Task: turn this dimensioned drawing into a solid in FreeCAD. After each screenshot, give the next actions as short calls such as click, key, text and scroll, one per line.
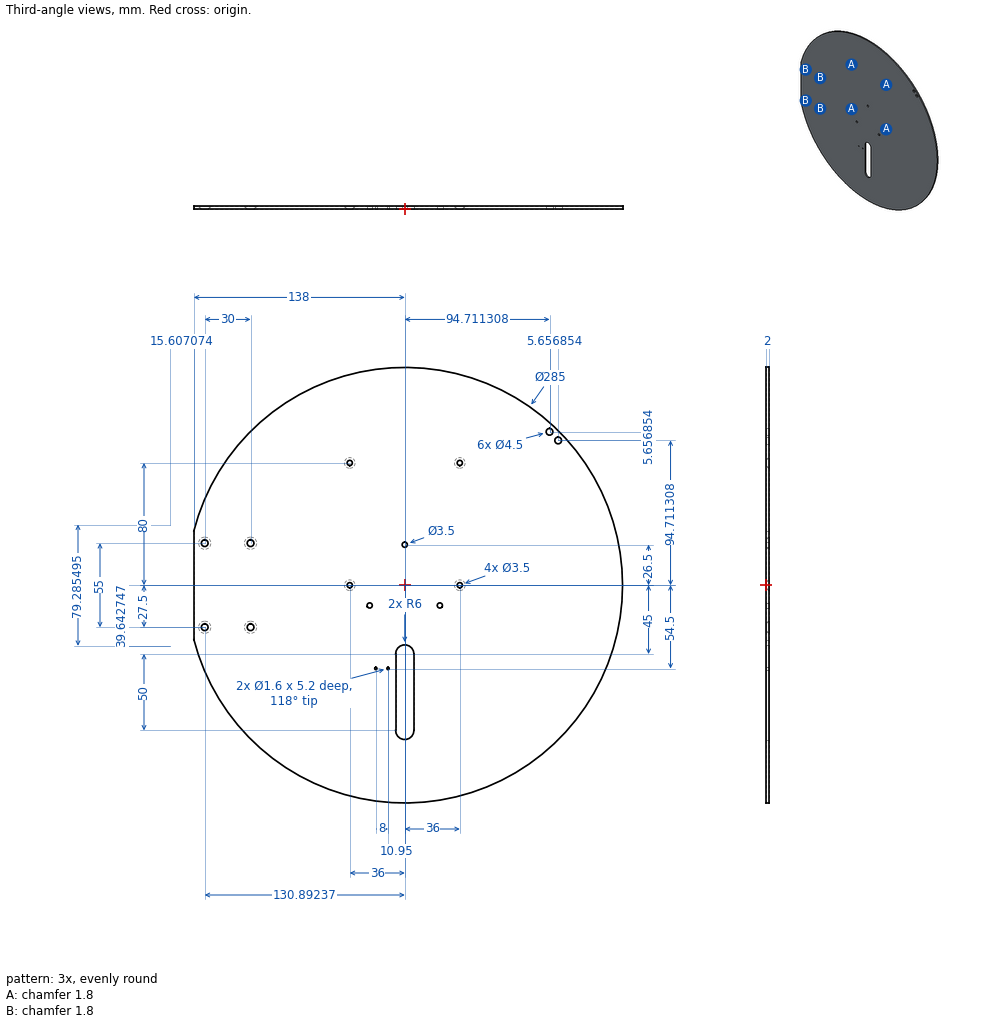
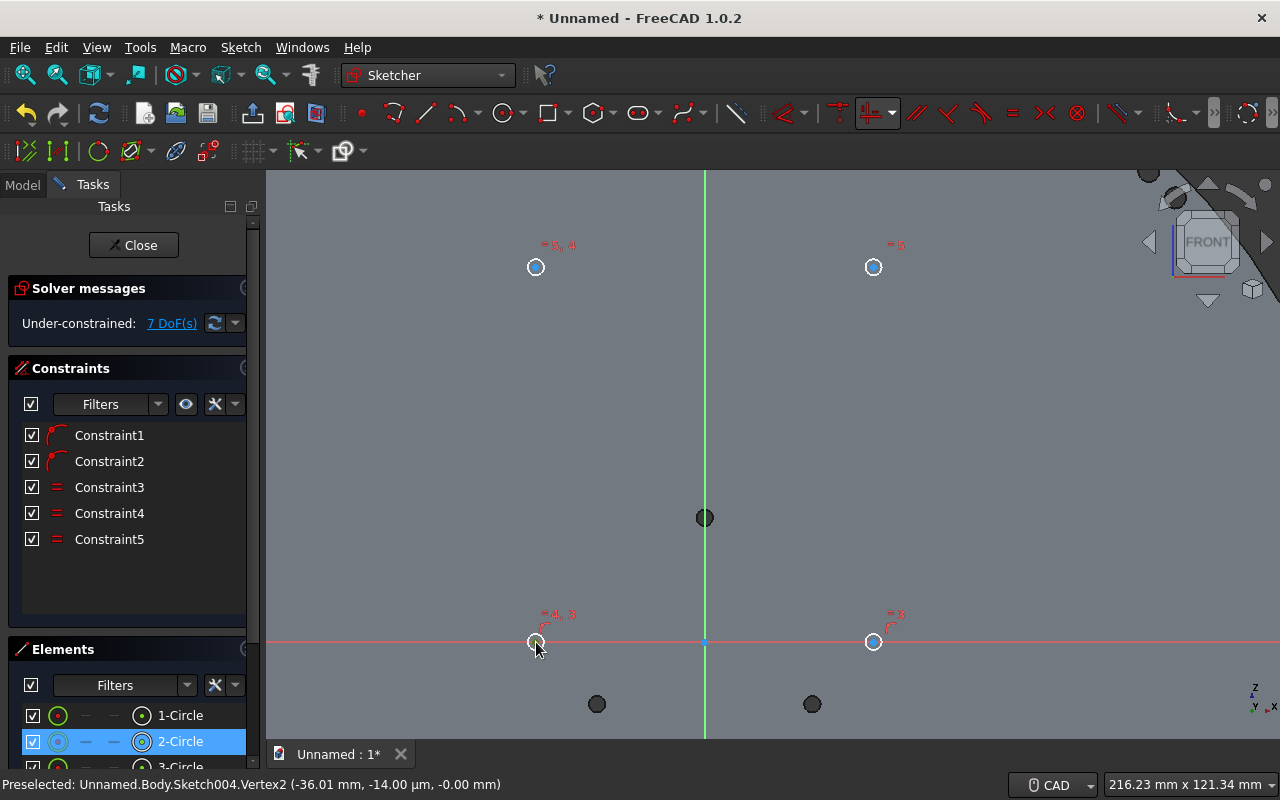
click(536, 267)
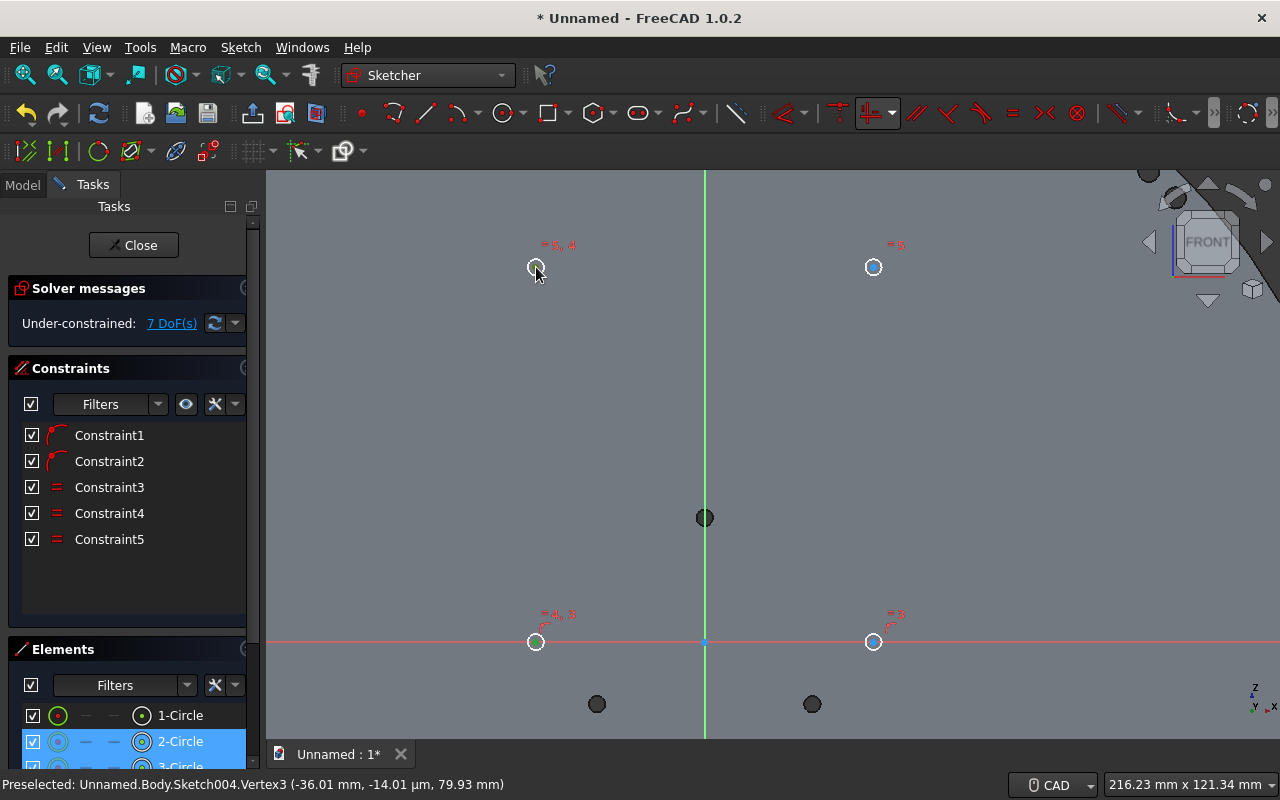
click(894, 114)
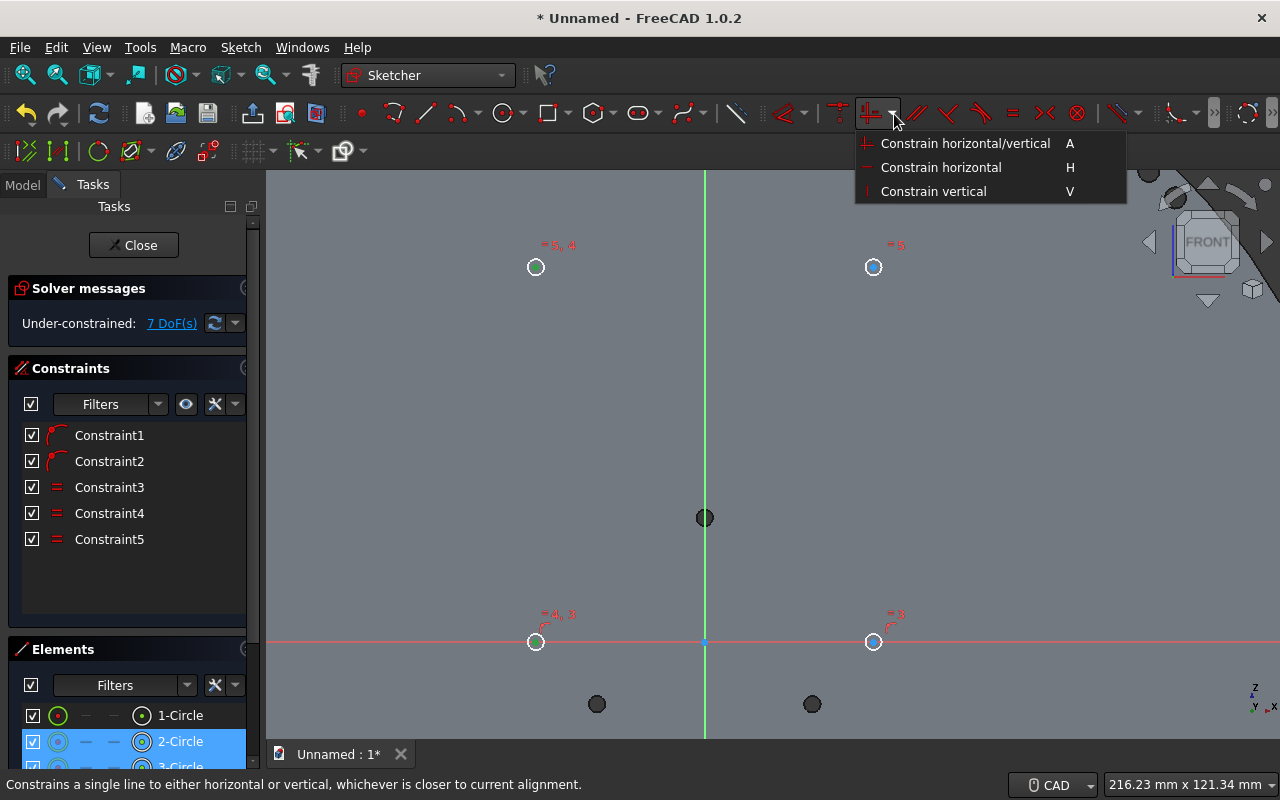
click(991, 191)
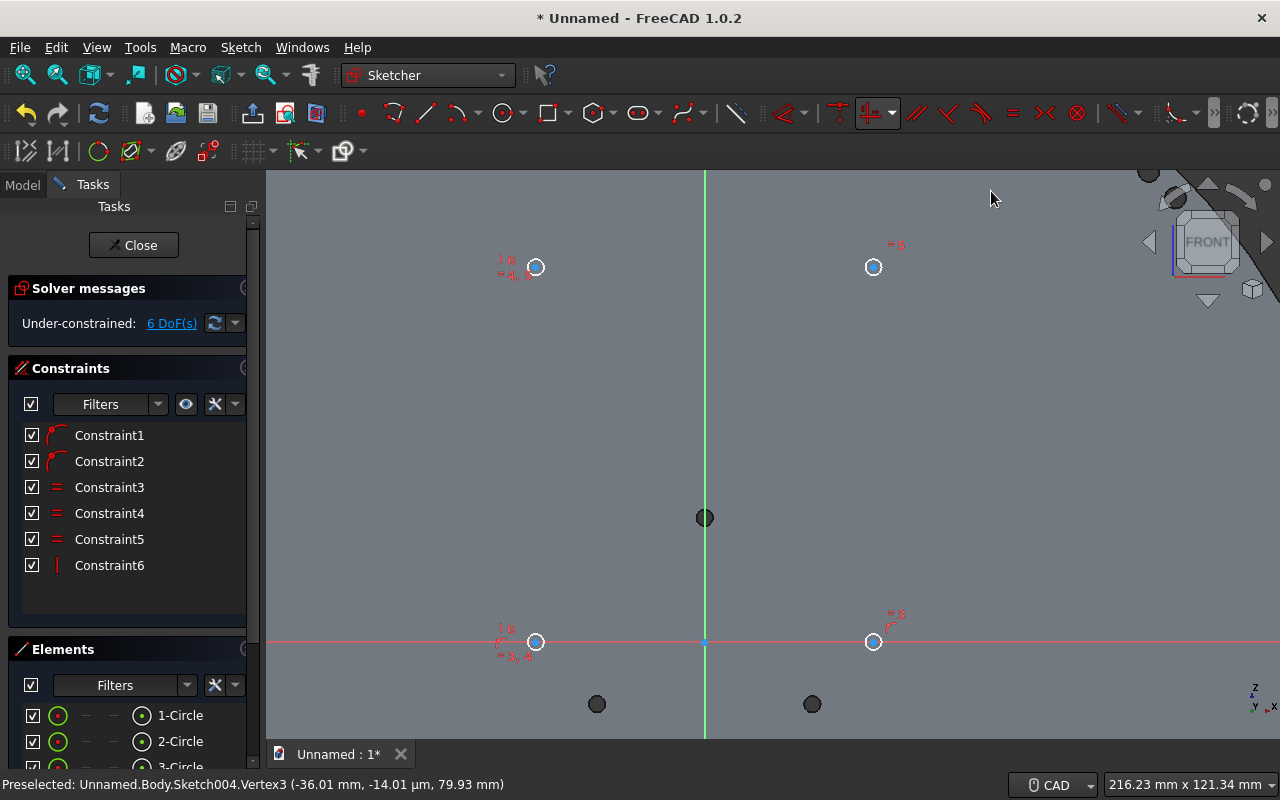
click(874, 642)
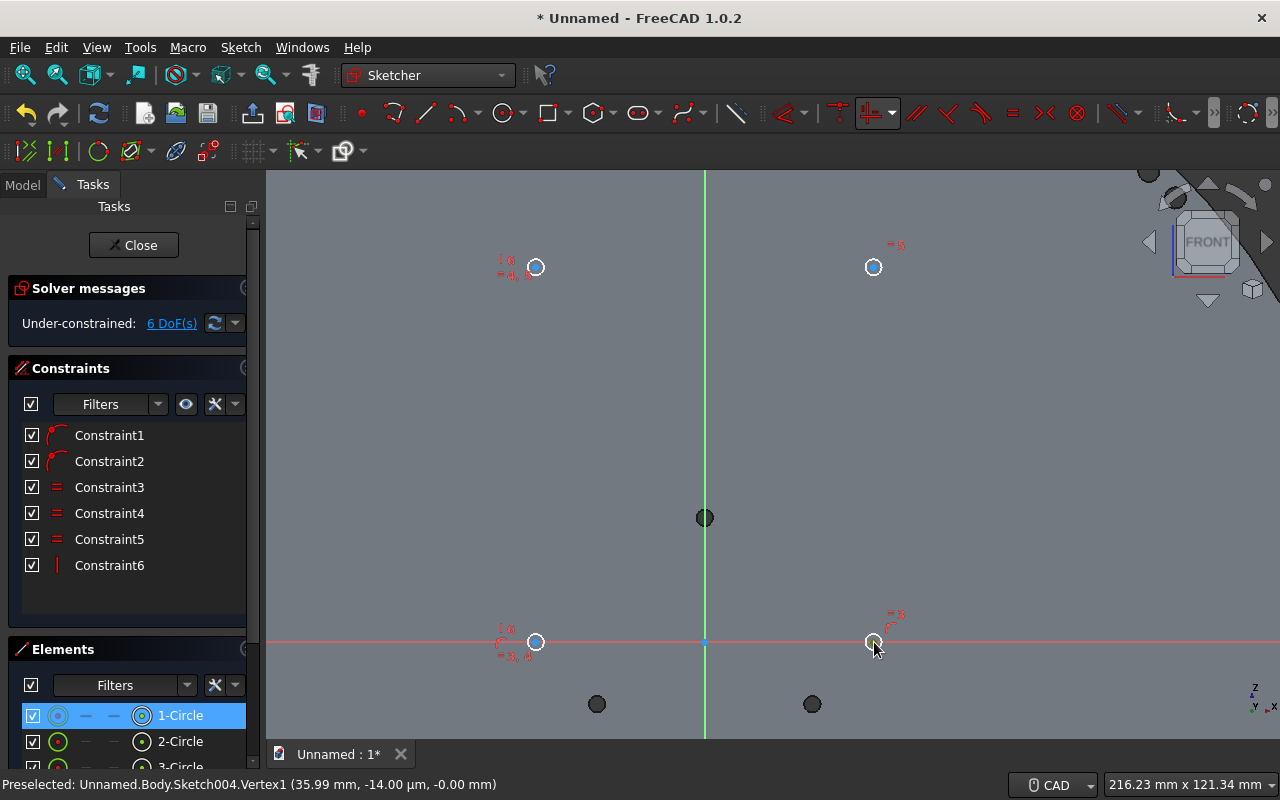
click(874, 267)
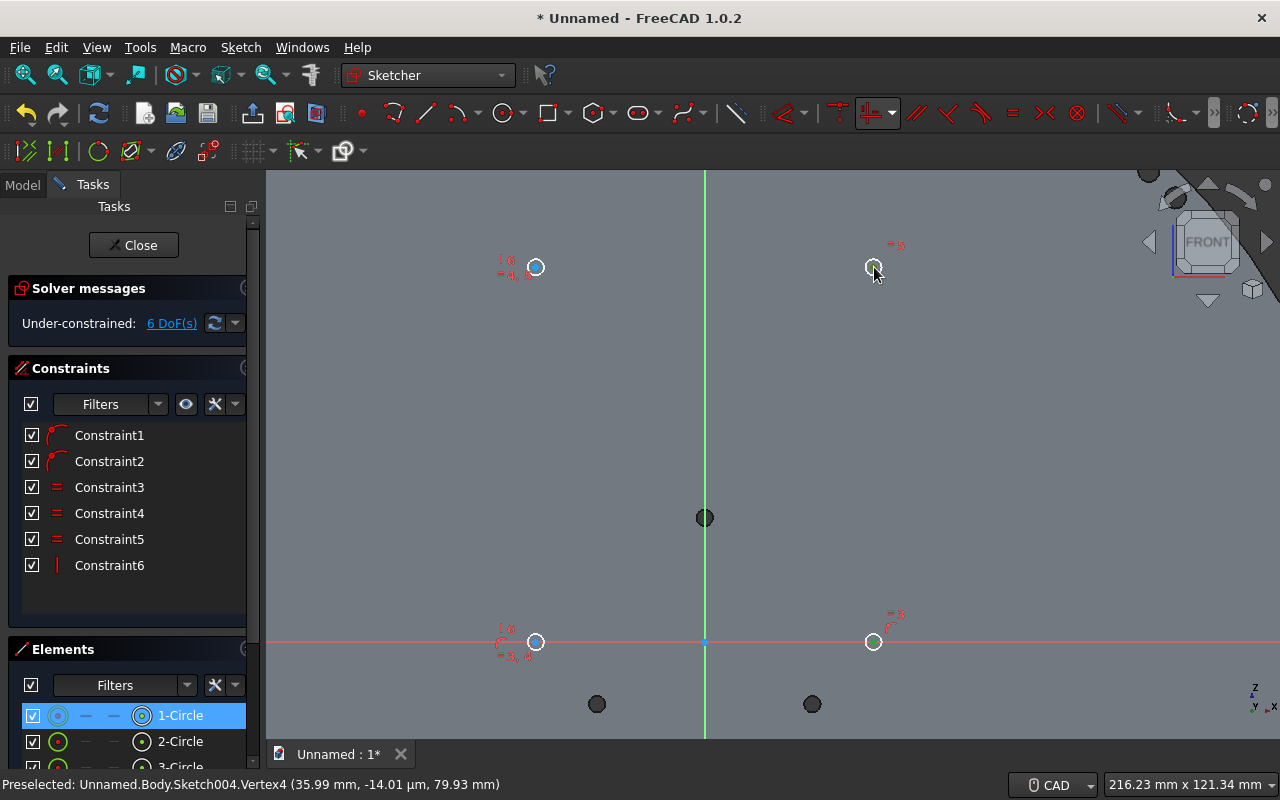
click(894, 114)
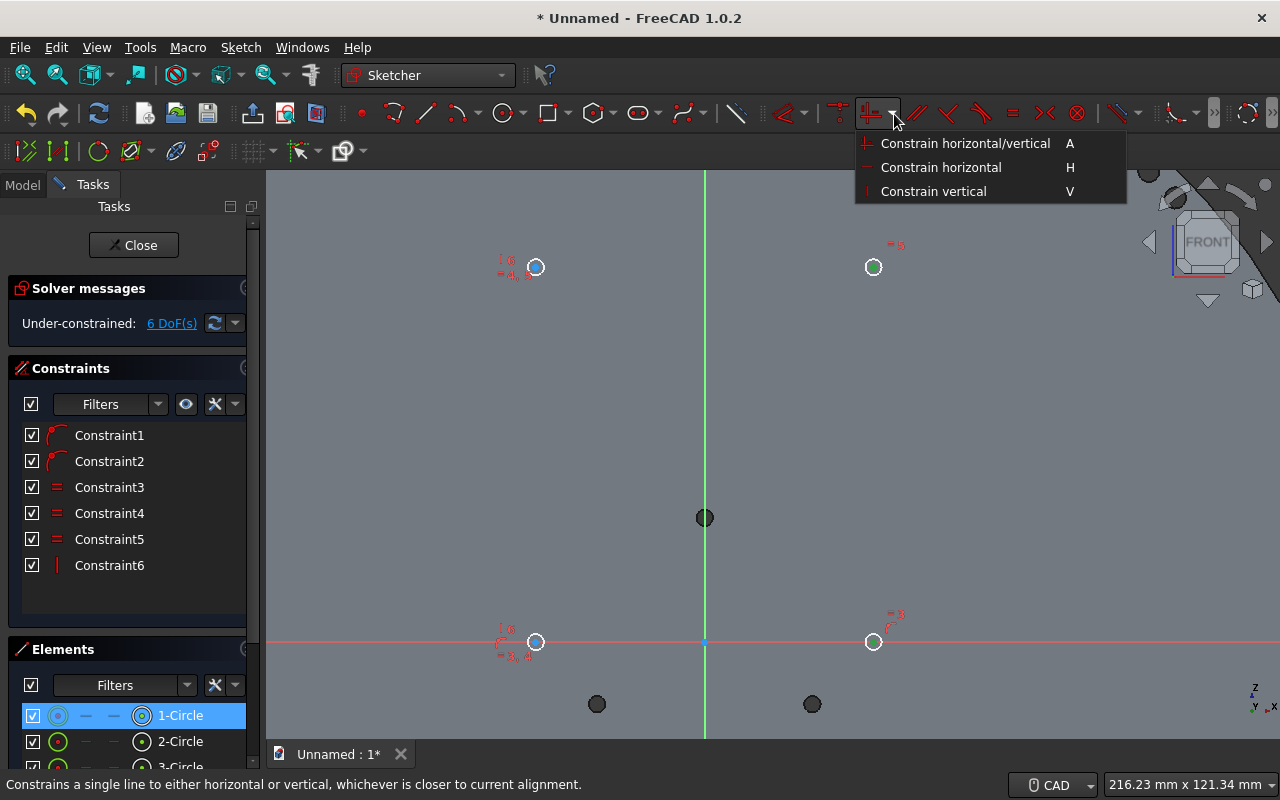
click(991, 191)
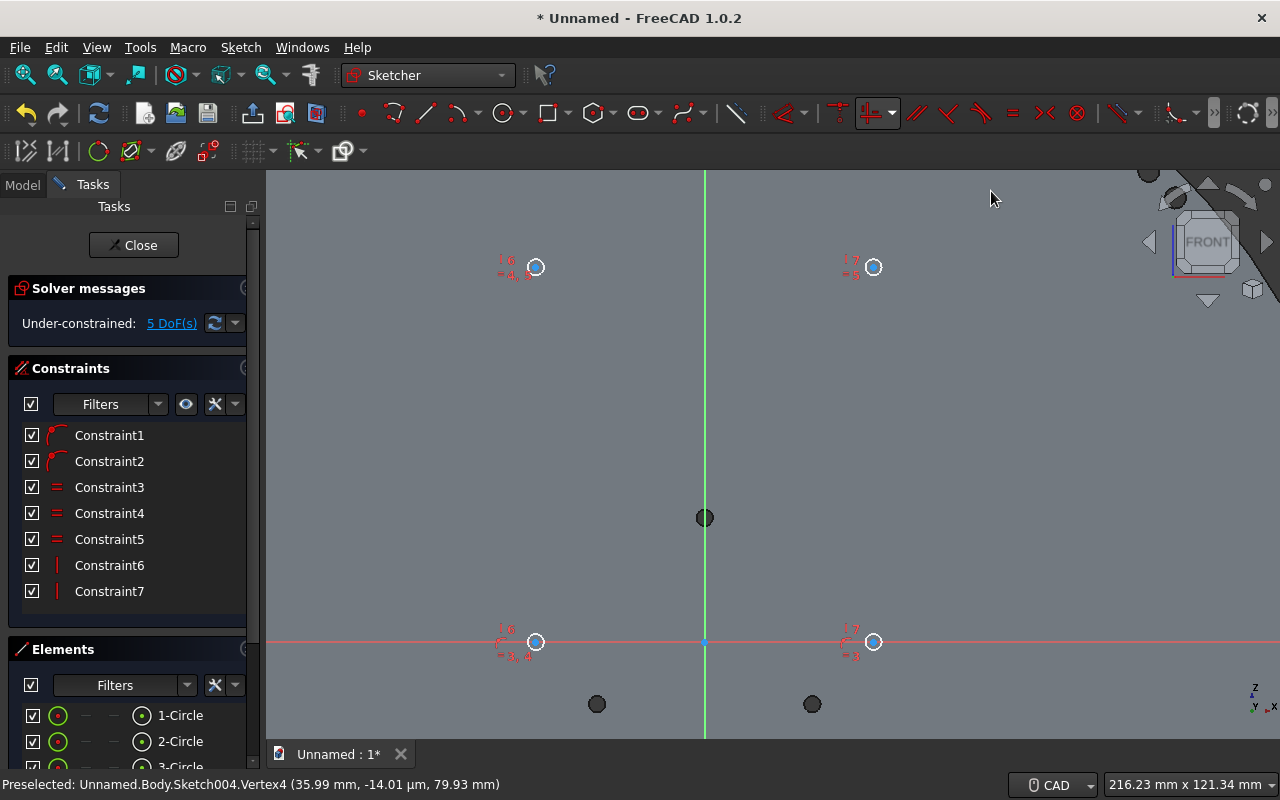
click(536, 267)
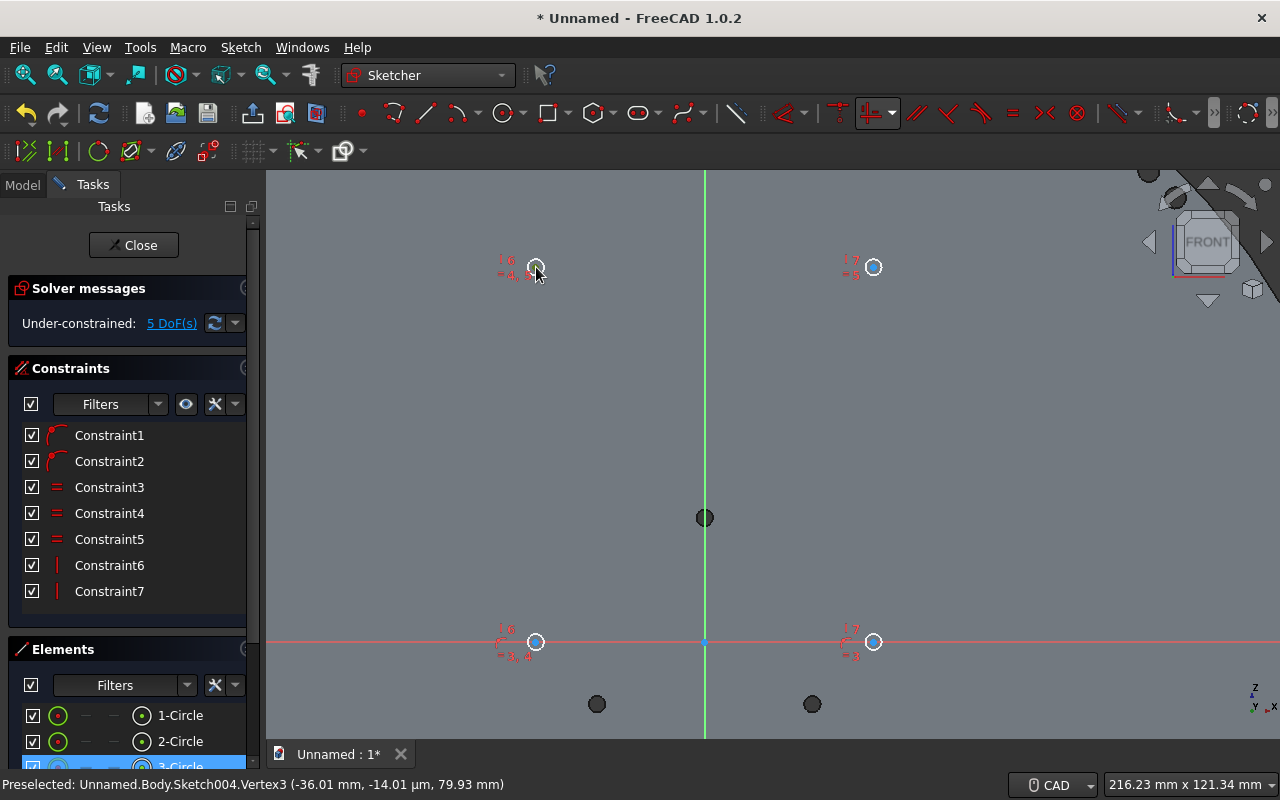
click(874, 267)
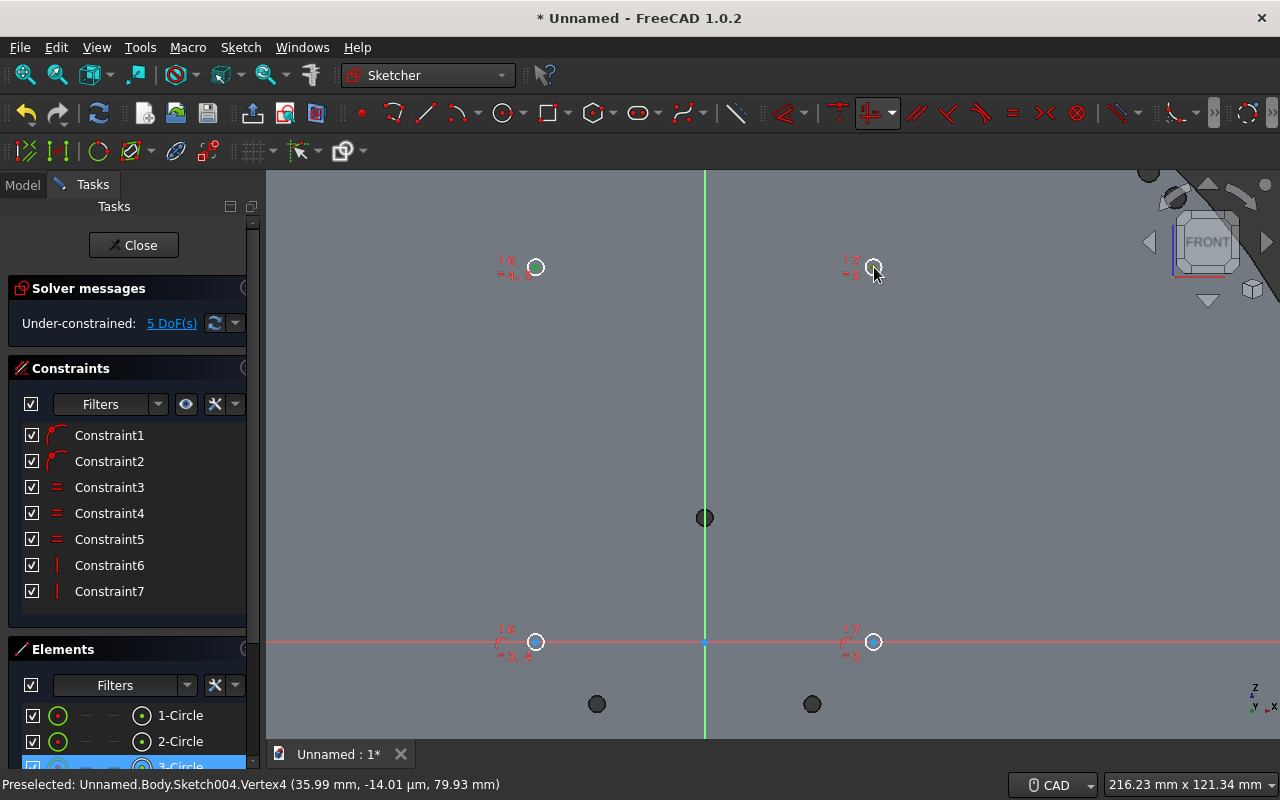
click(894, 114)